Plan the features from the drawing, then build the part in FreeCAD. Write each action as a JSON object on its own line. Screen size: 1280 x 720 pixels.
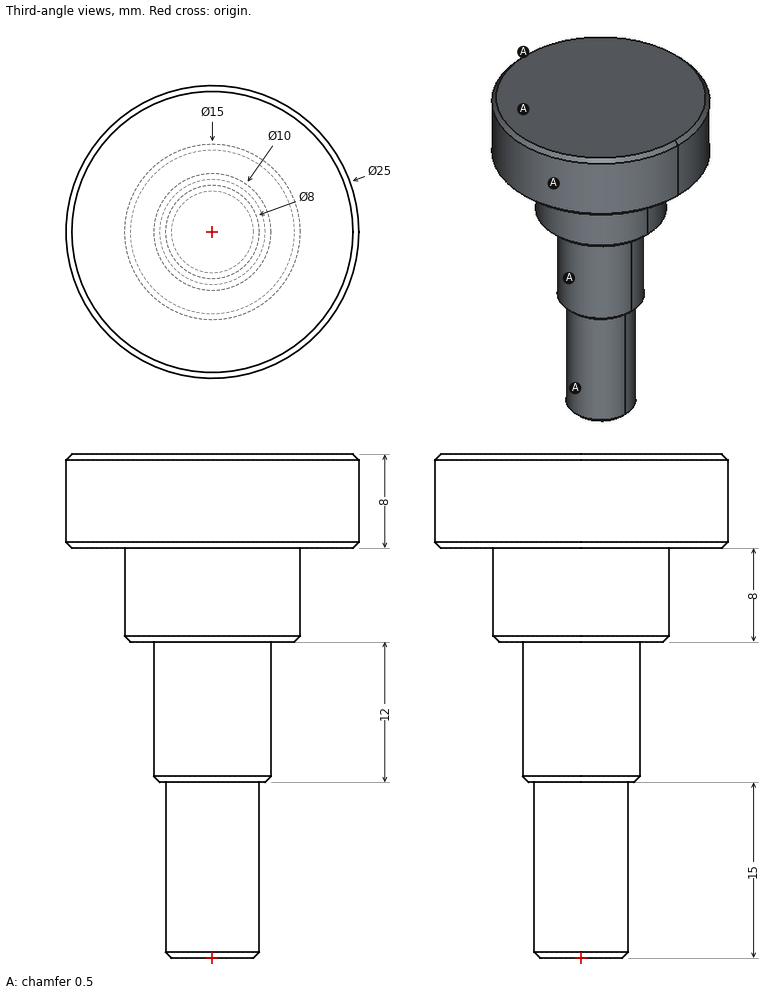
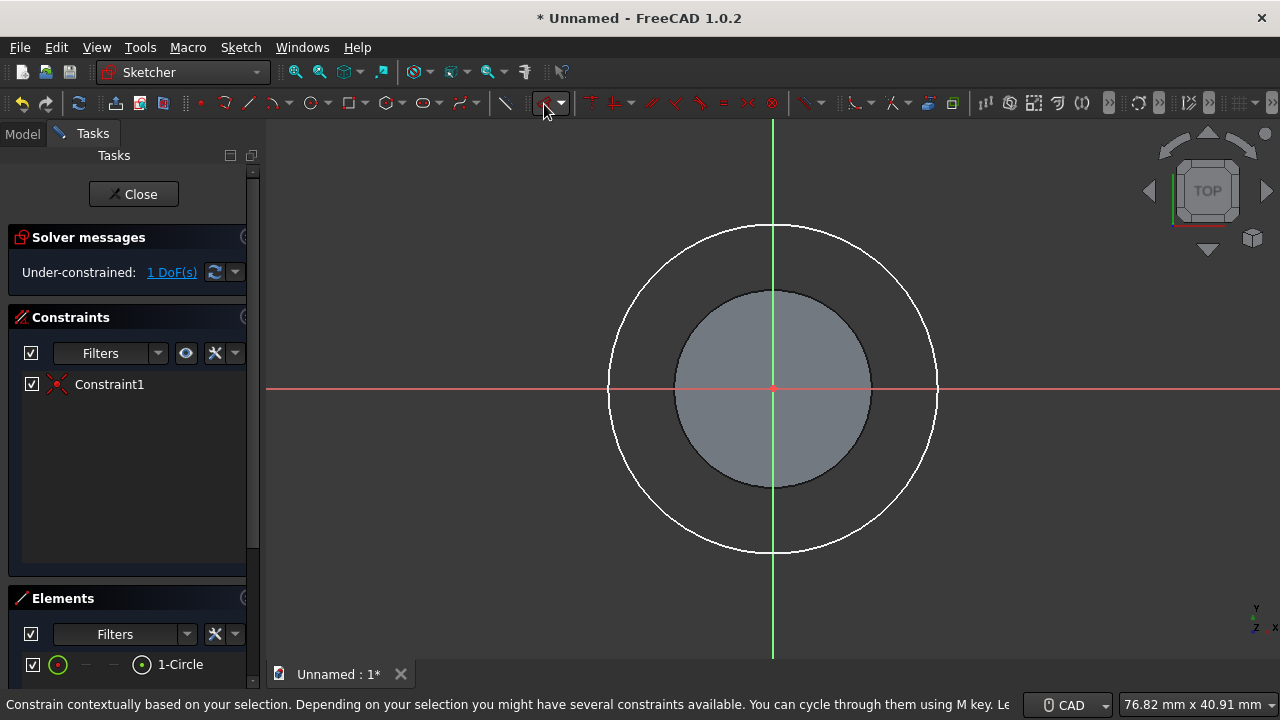
{"action": "left_click", "coordinate": [889, 272]}
{"action": "left_click", "coordinate": [912, 249]}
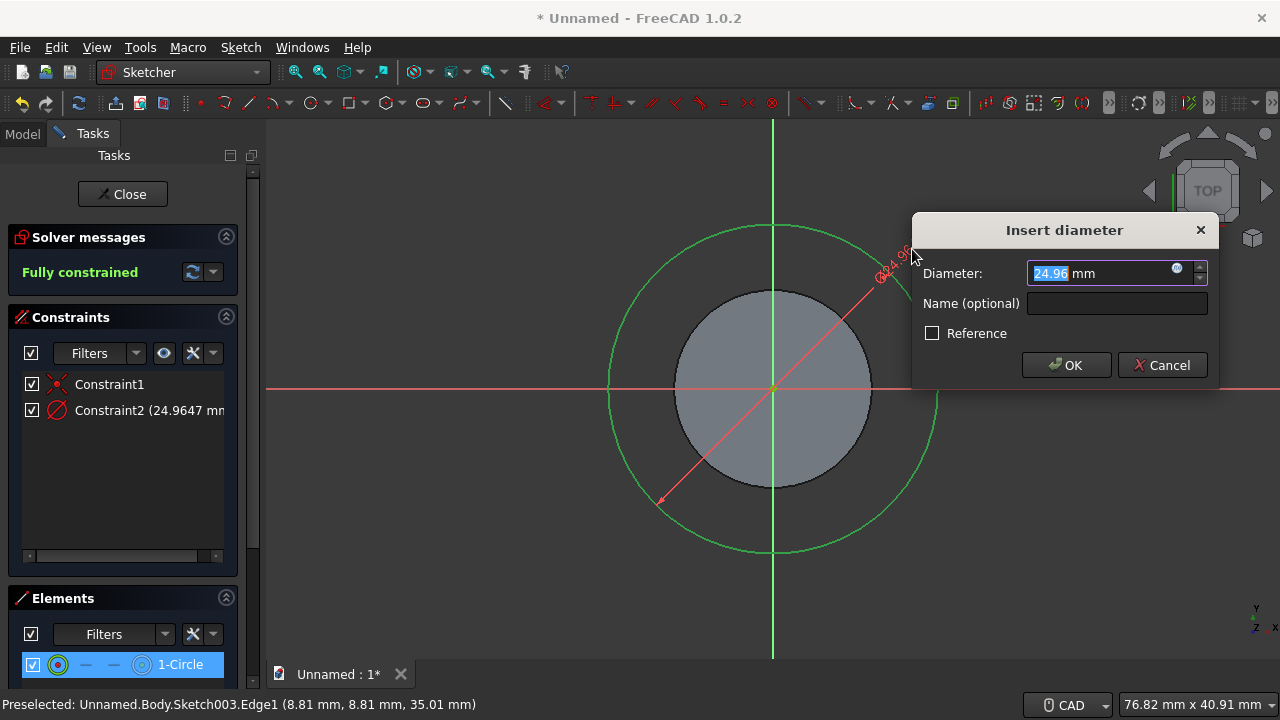
{"action": "type", "text": "25"}
{"action": "key", "text": "Return"}
{"action": "key", "text": "Escape"}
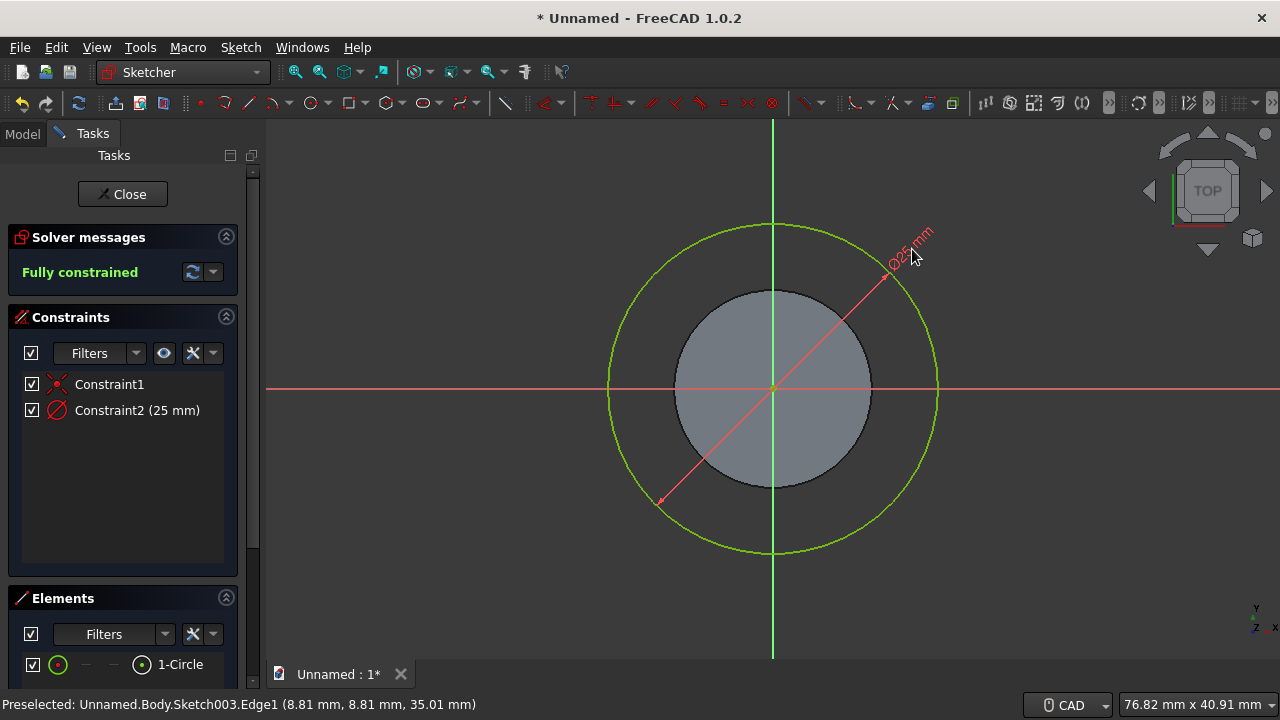
{"action": "left_click", "coordinate": [123, 194]}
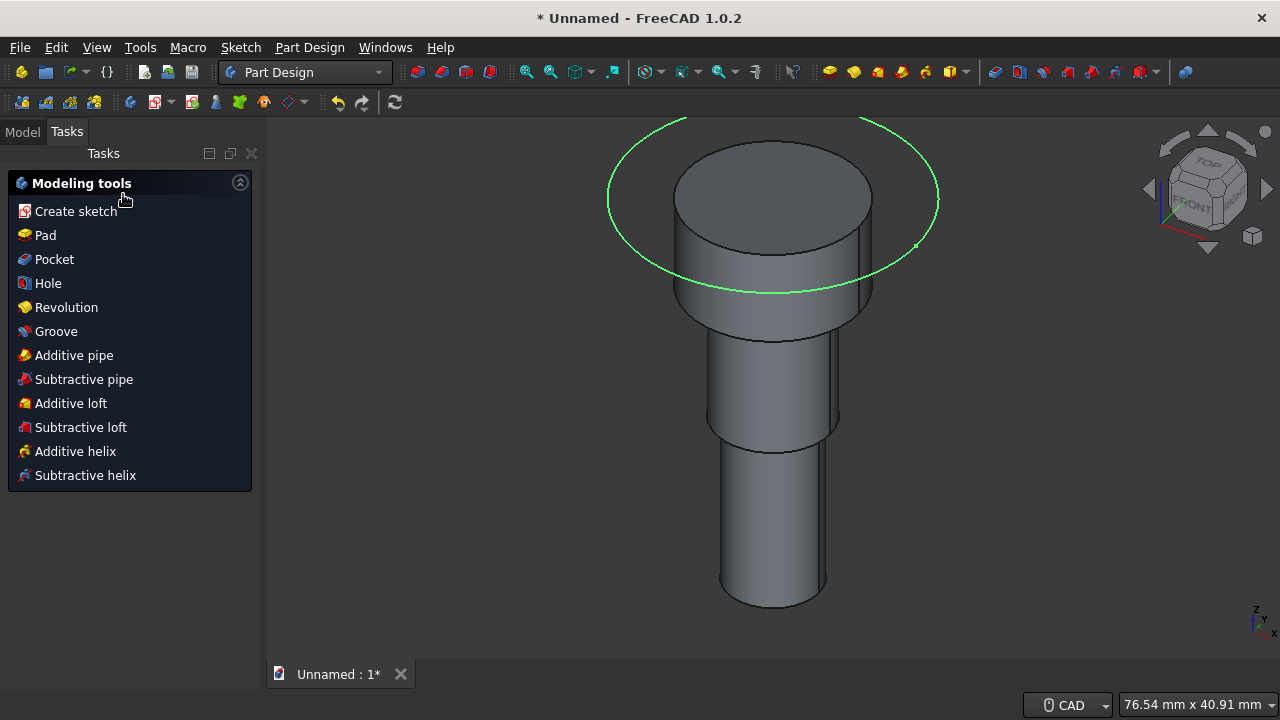
{"action": "left_click", "coordinate": [830, 72]}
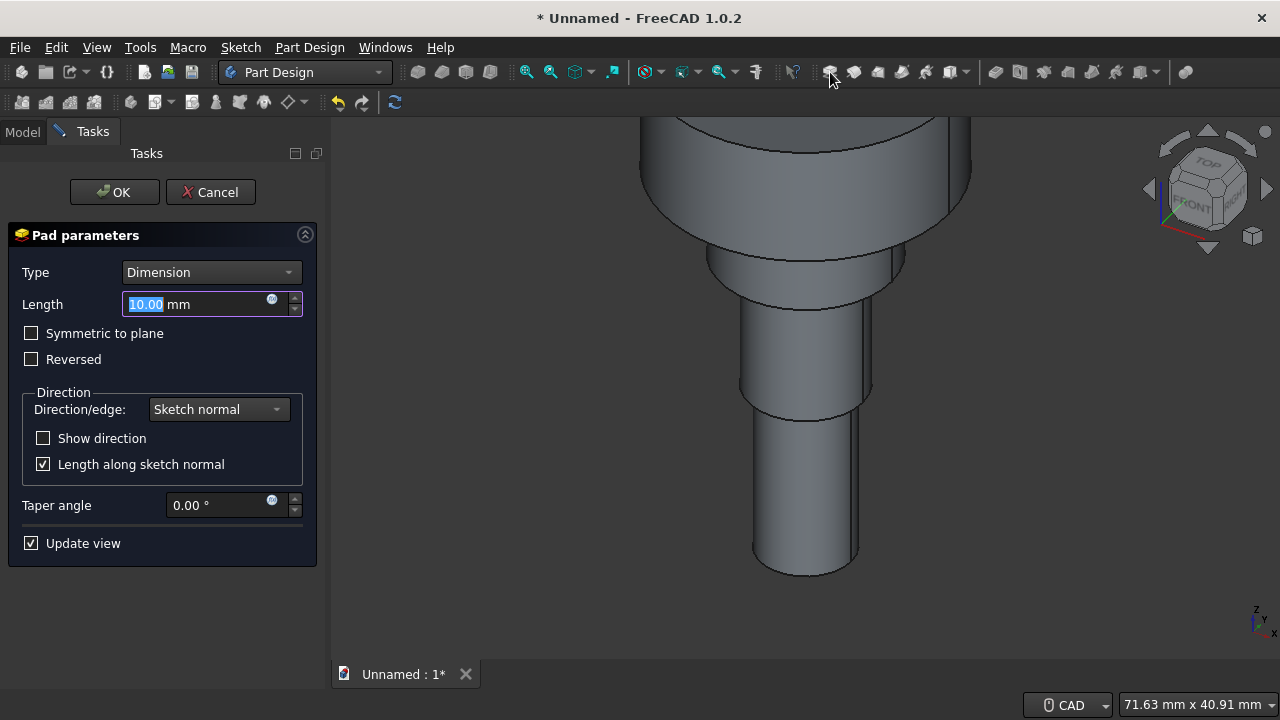
{"action": "type", "text": "8"}
{"action": "key", "text": "Tab"}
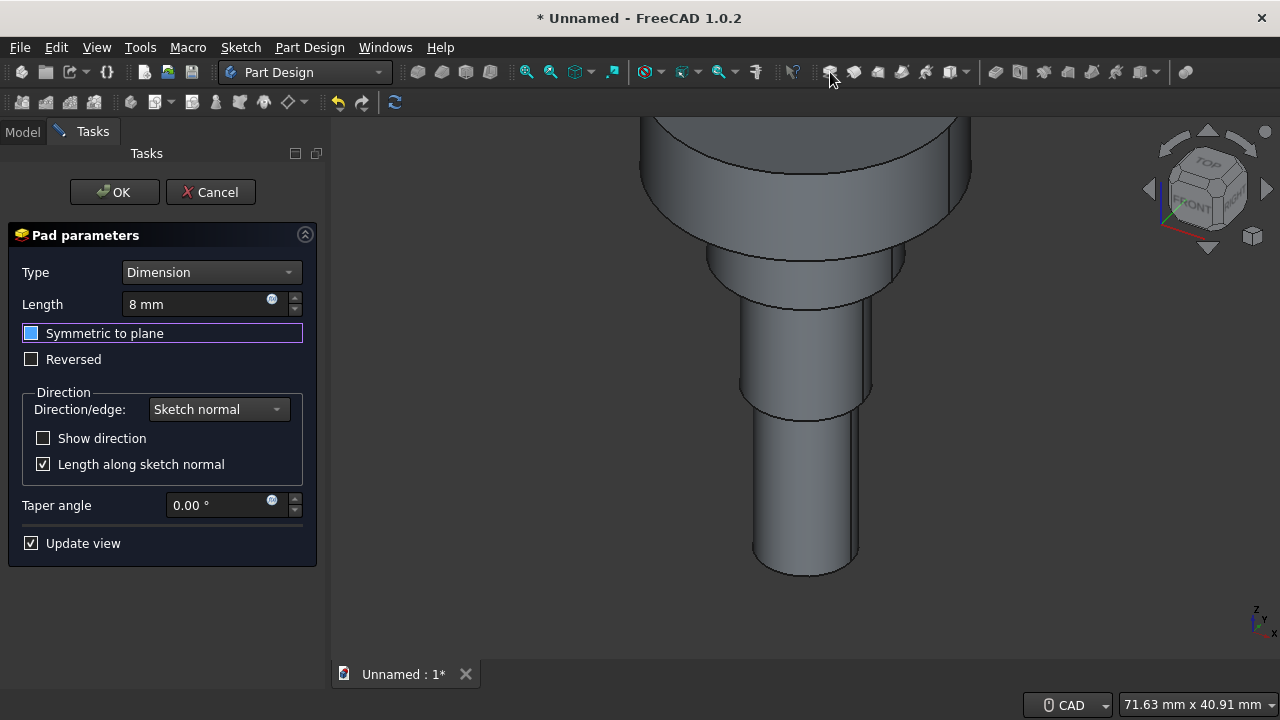
{"action": "left_click", "coordinate": [115, 192]}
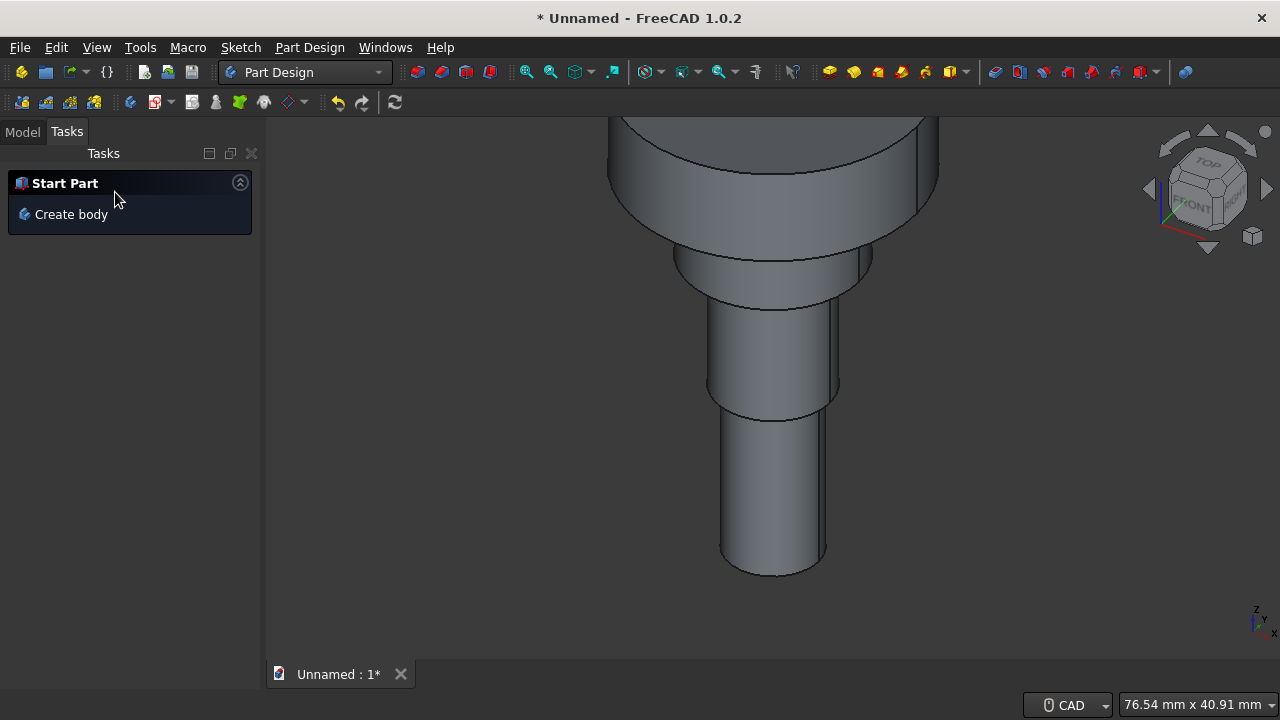
{"action": "left_click", "coordinate": [528, 72]}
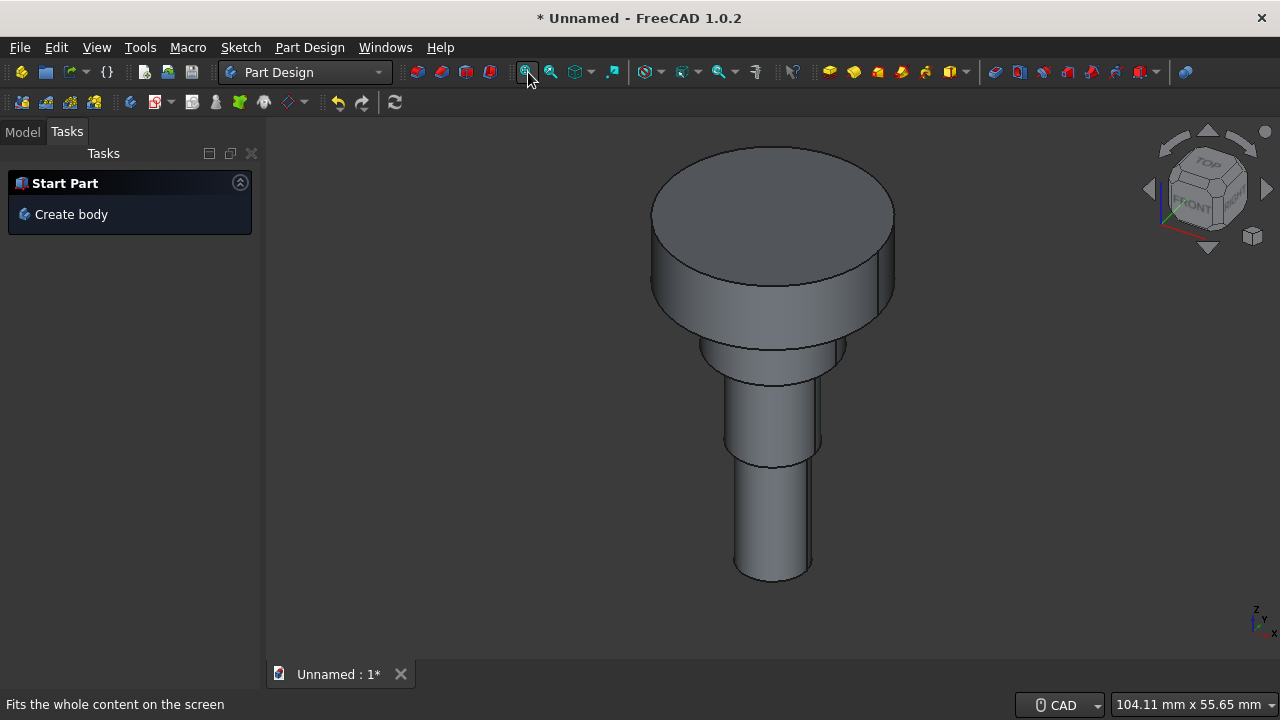
{"action": "left_click", "coordinate": [652, 223]}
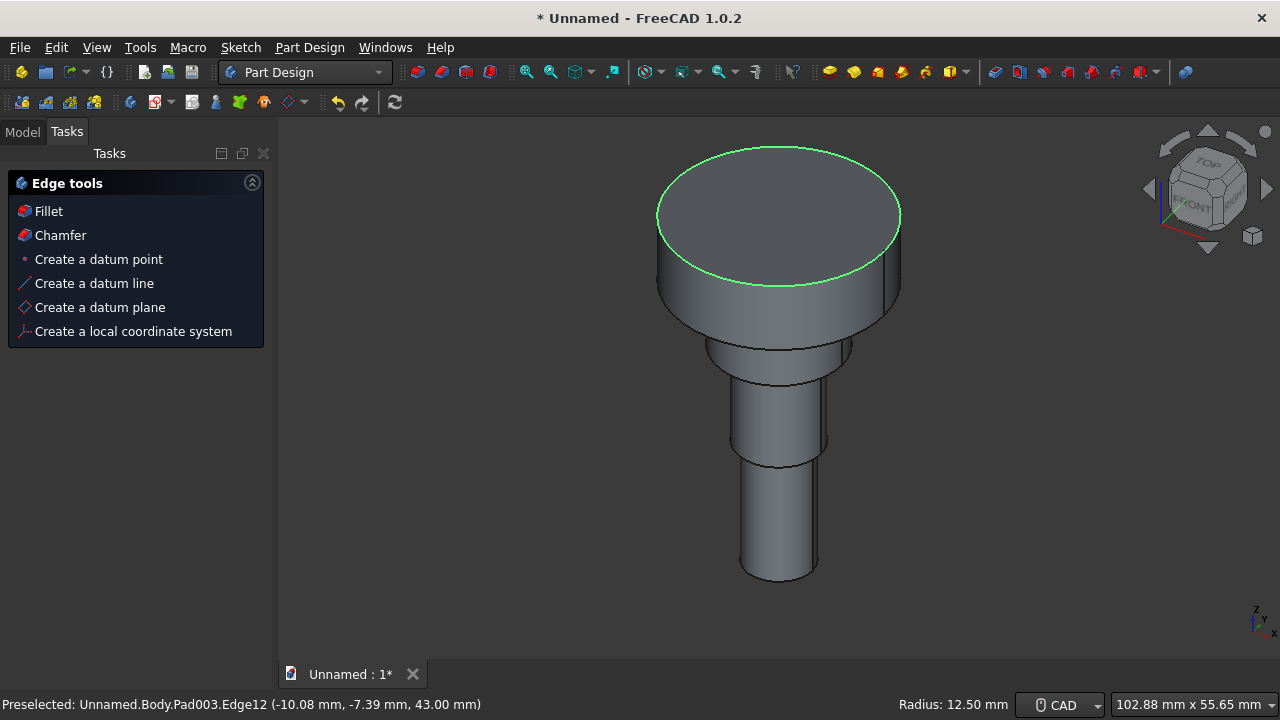
{"action": "left_click", "coordinate": [743, 458], "text": "ctrl"}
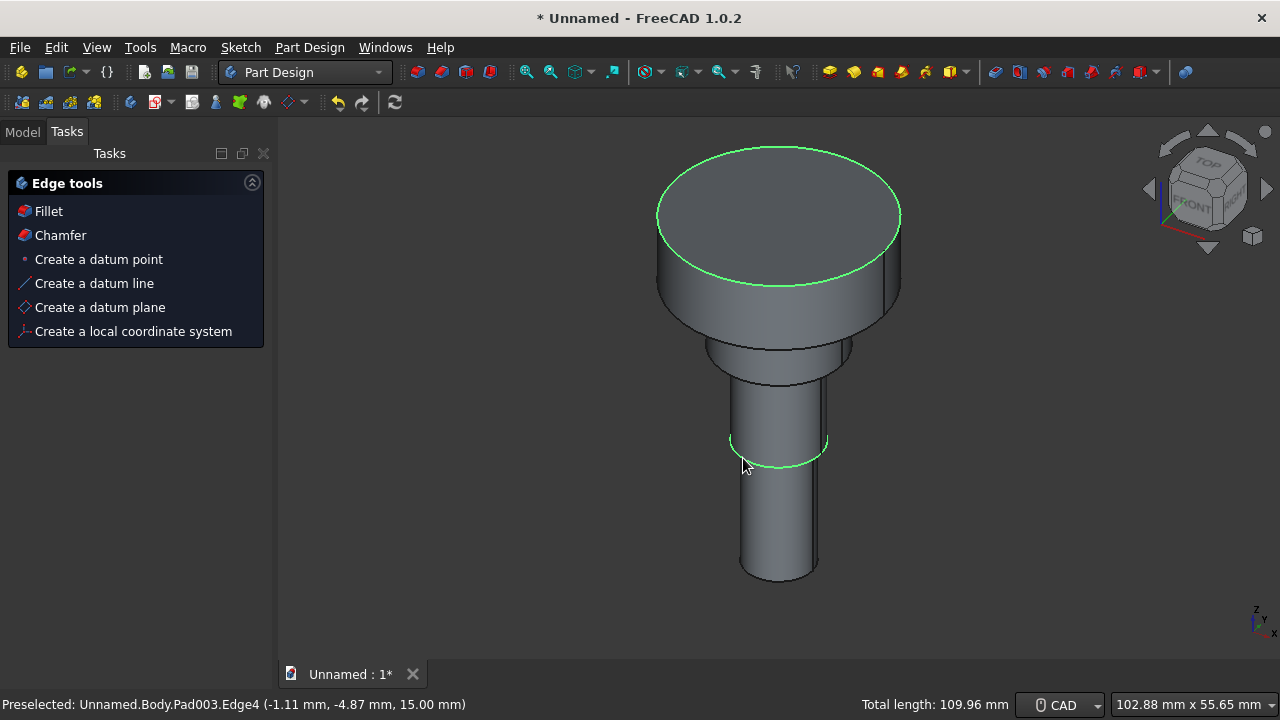
{"action": "key", "text": "0"}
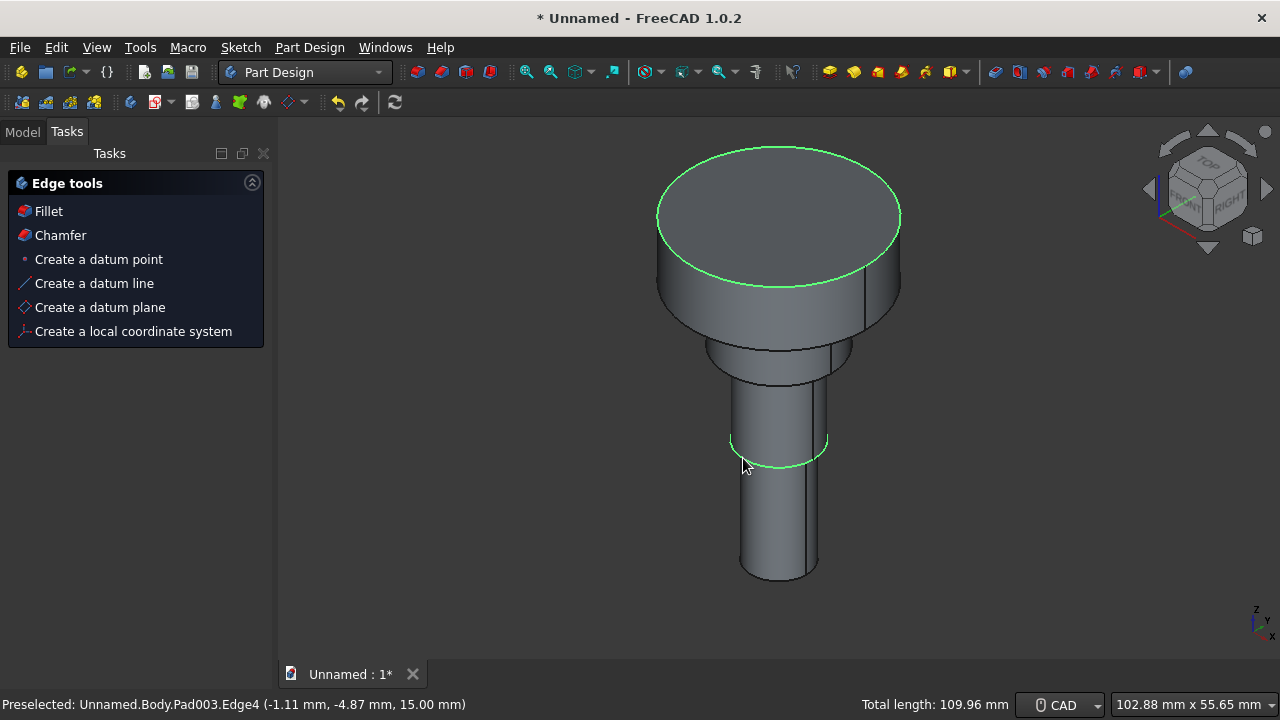
{"action": "key", "text": "2"}